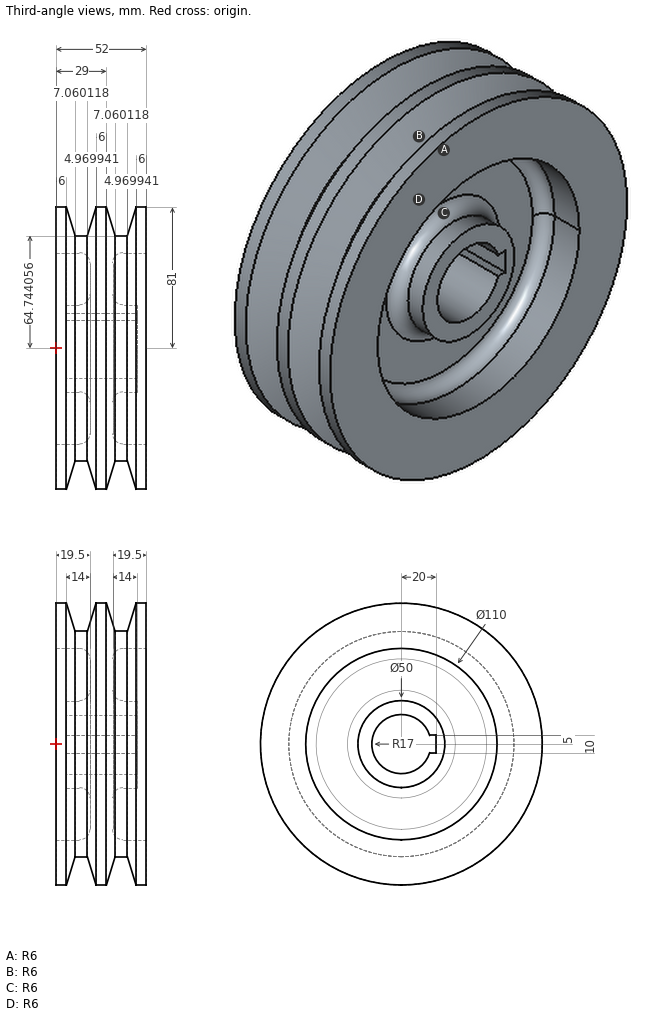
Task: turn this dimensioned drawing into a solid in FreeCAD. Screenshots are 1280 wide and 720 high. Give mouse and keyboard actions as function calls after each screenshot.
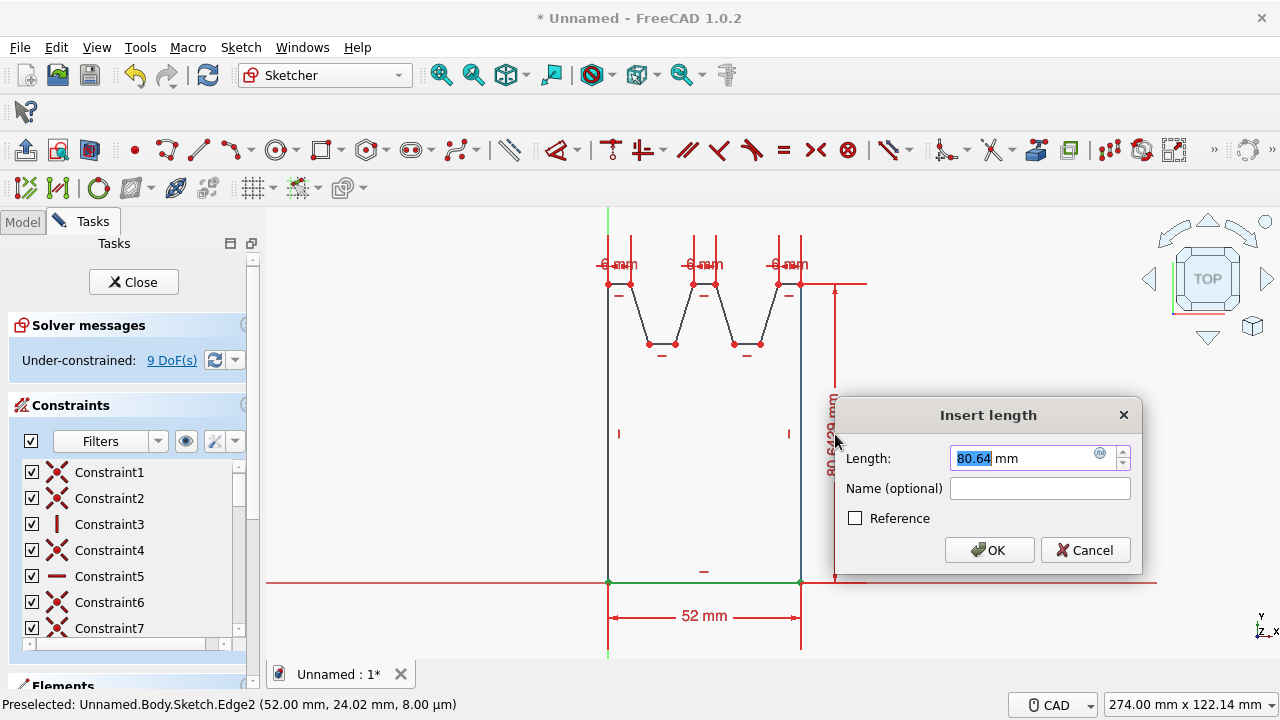
text(81)
key(Return)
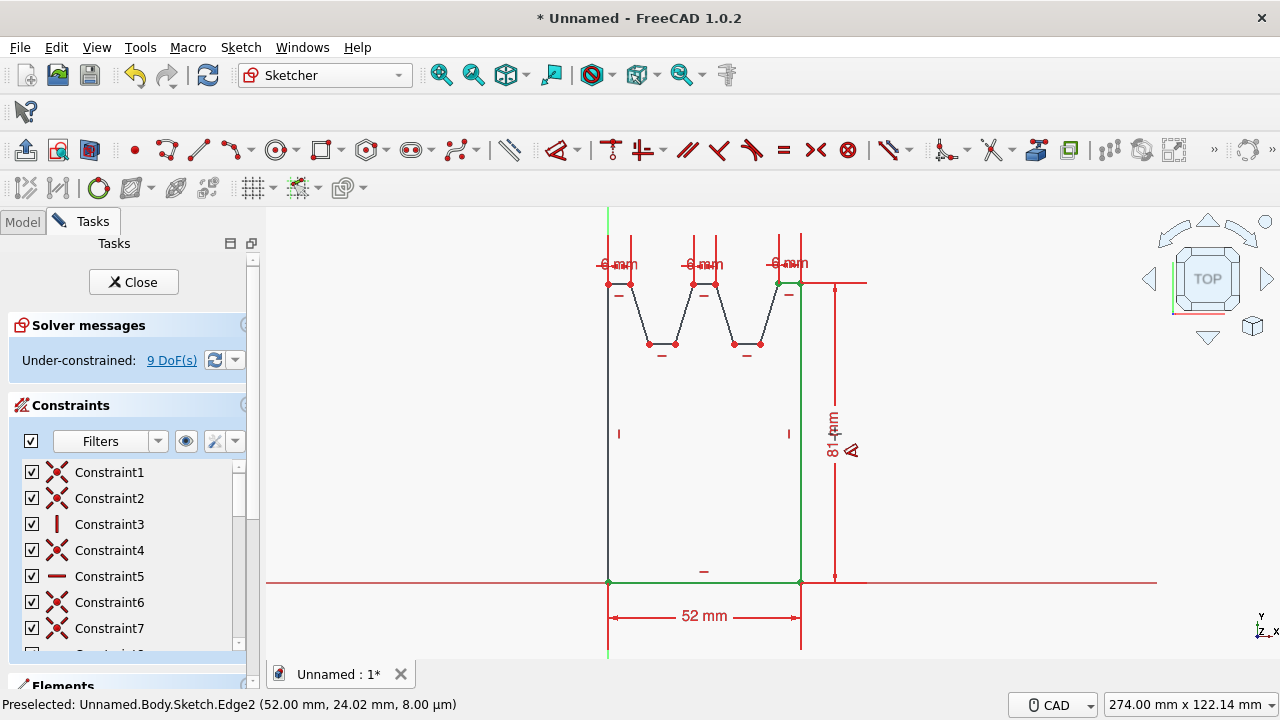
click(608, 374)
click(574, 434)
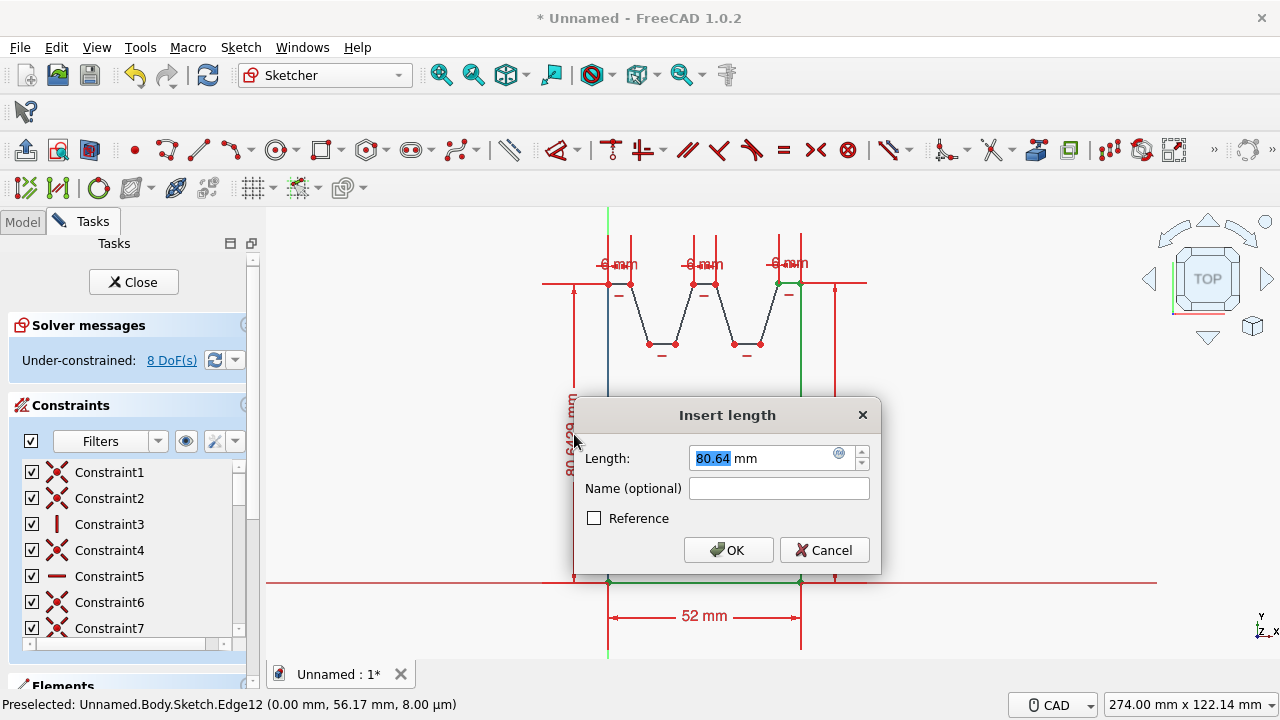
text(81)
key(Return)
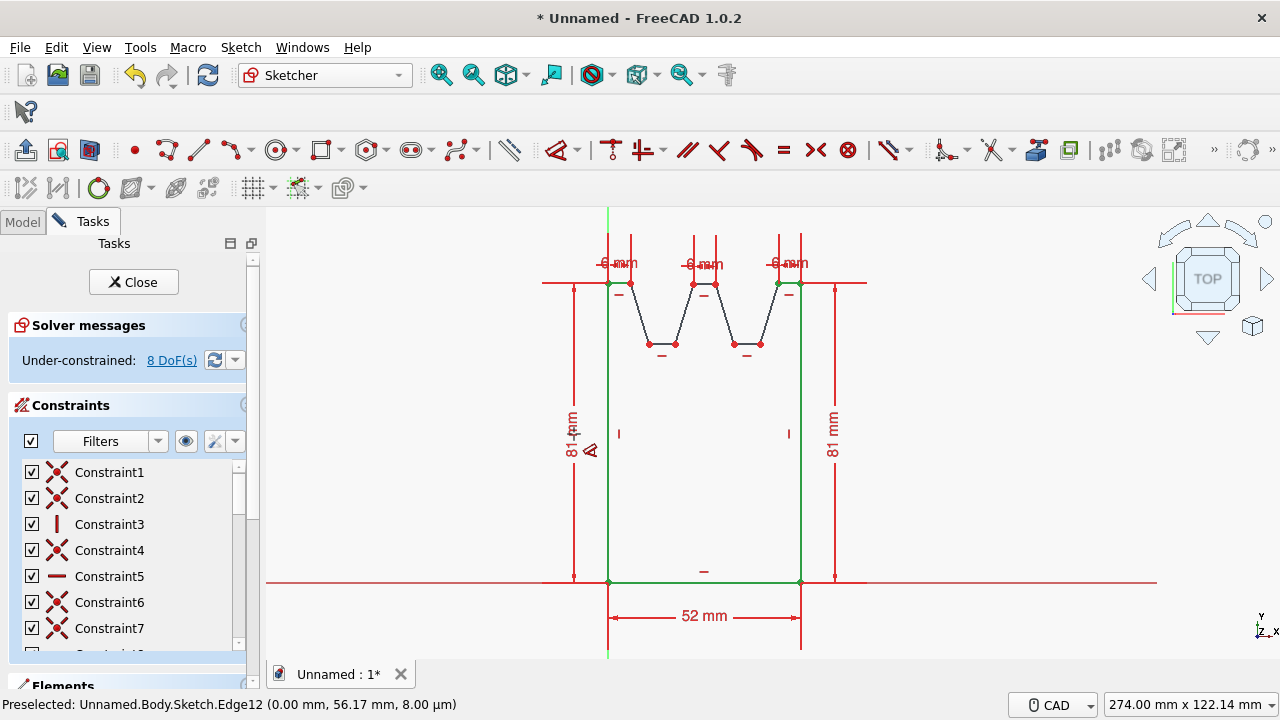
click(716, 284)
click(624, 617)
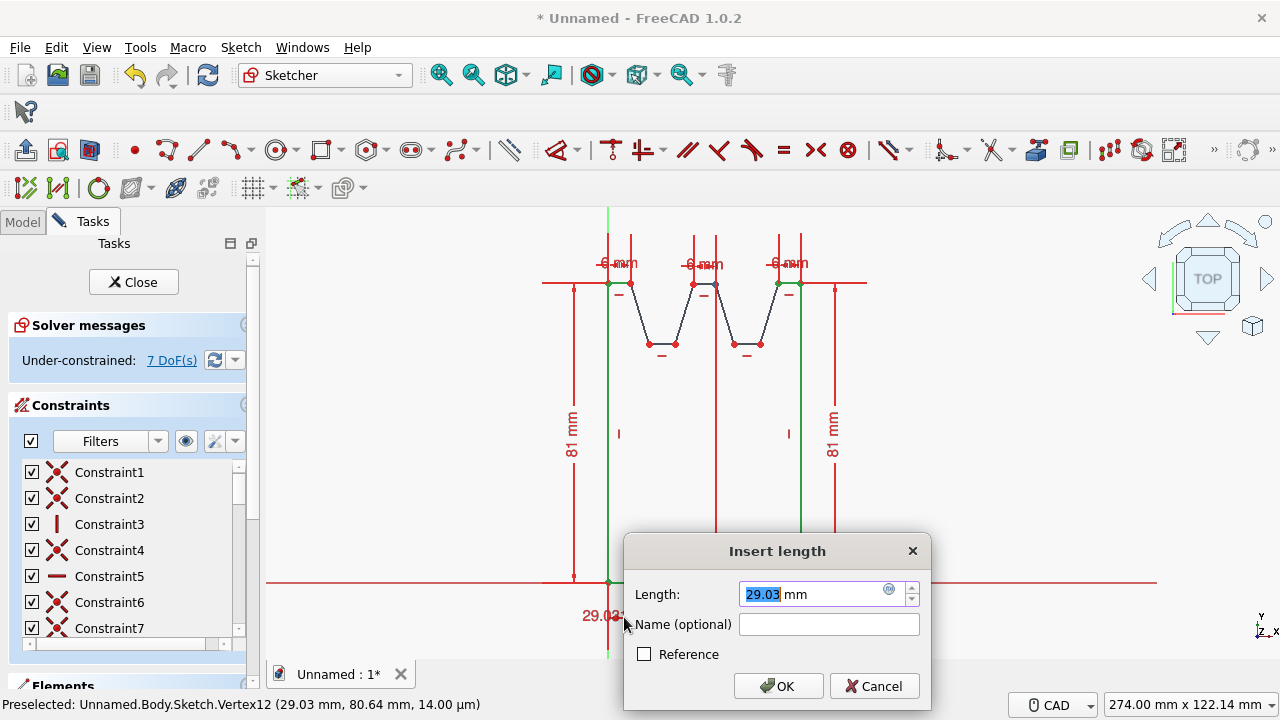
text(29)
key(Return)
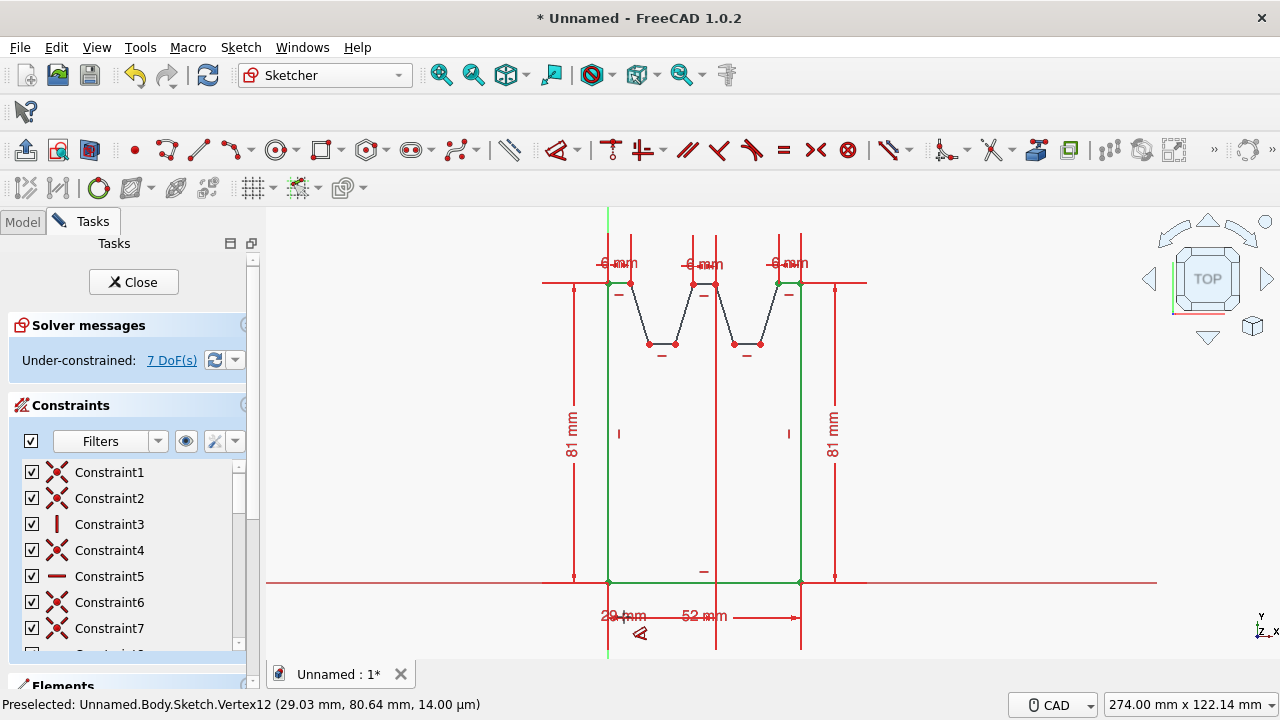
click(716, 284)
click(574, 365)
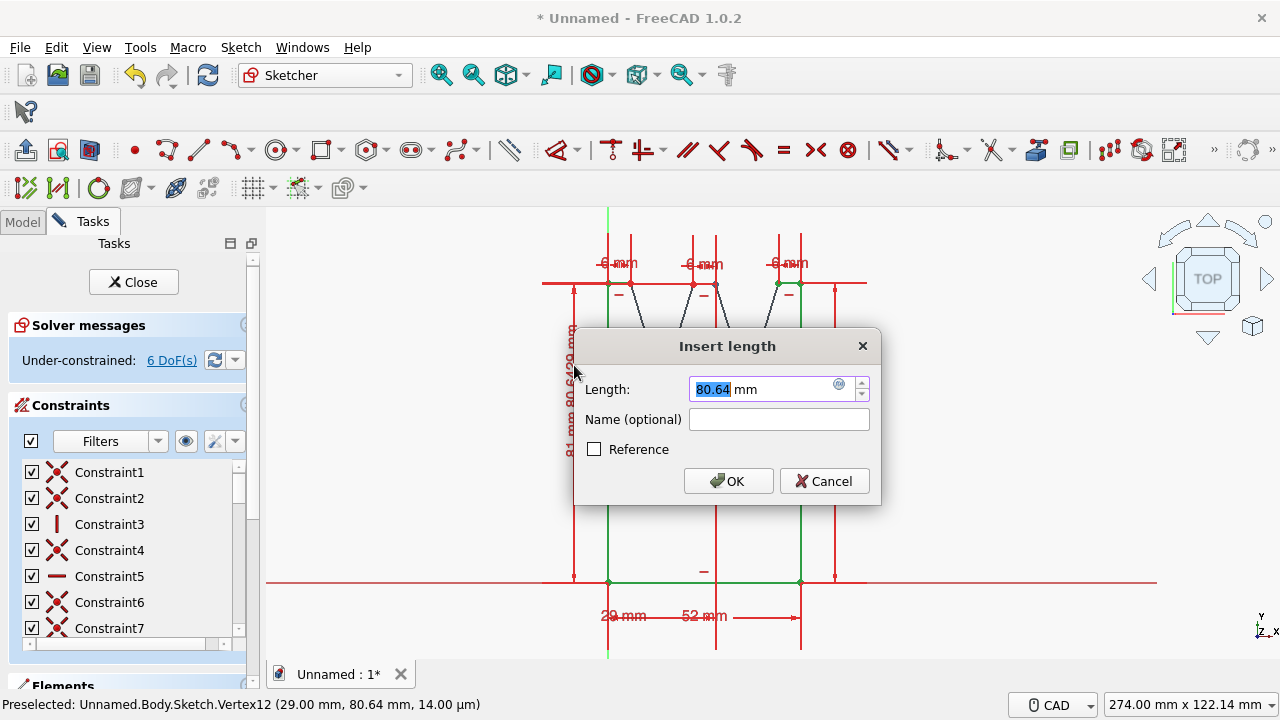
text(81)
key(Return)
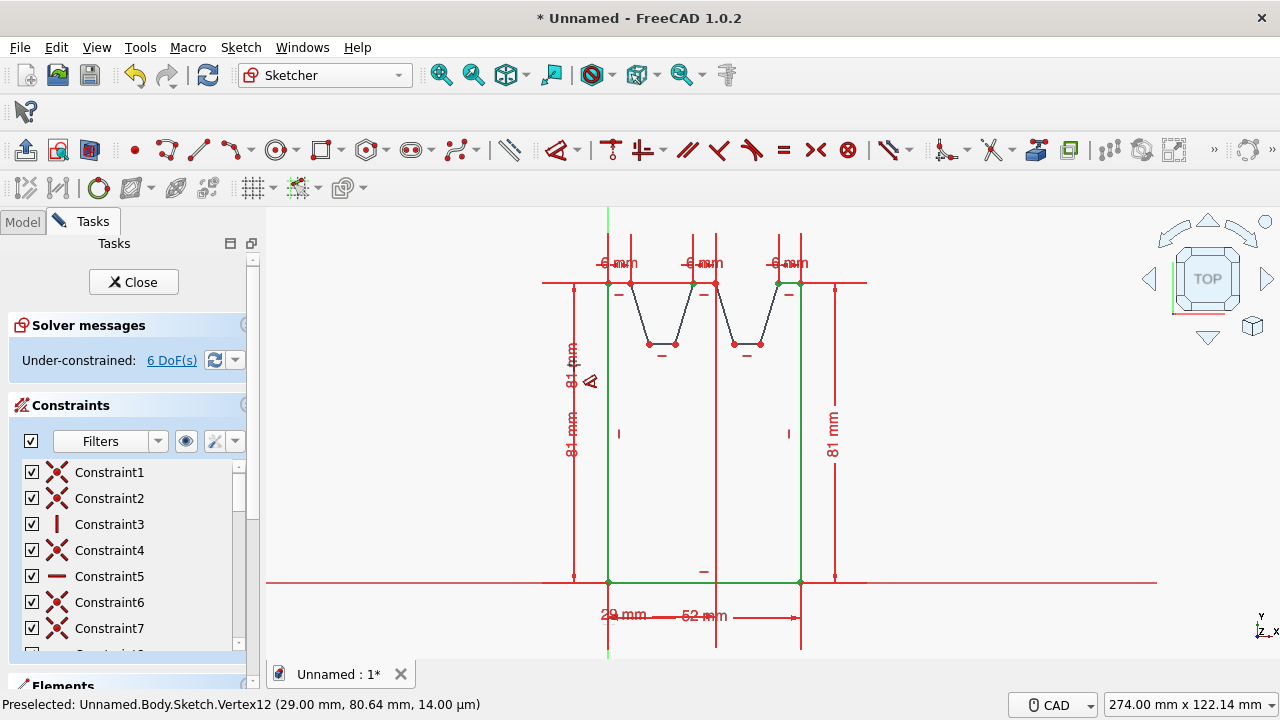
scroll(750, 344, up, 3)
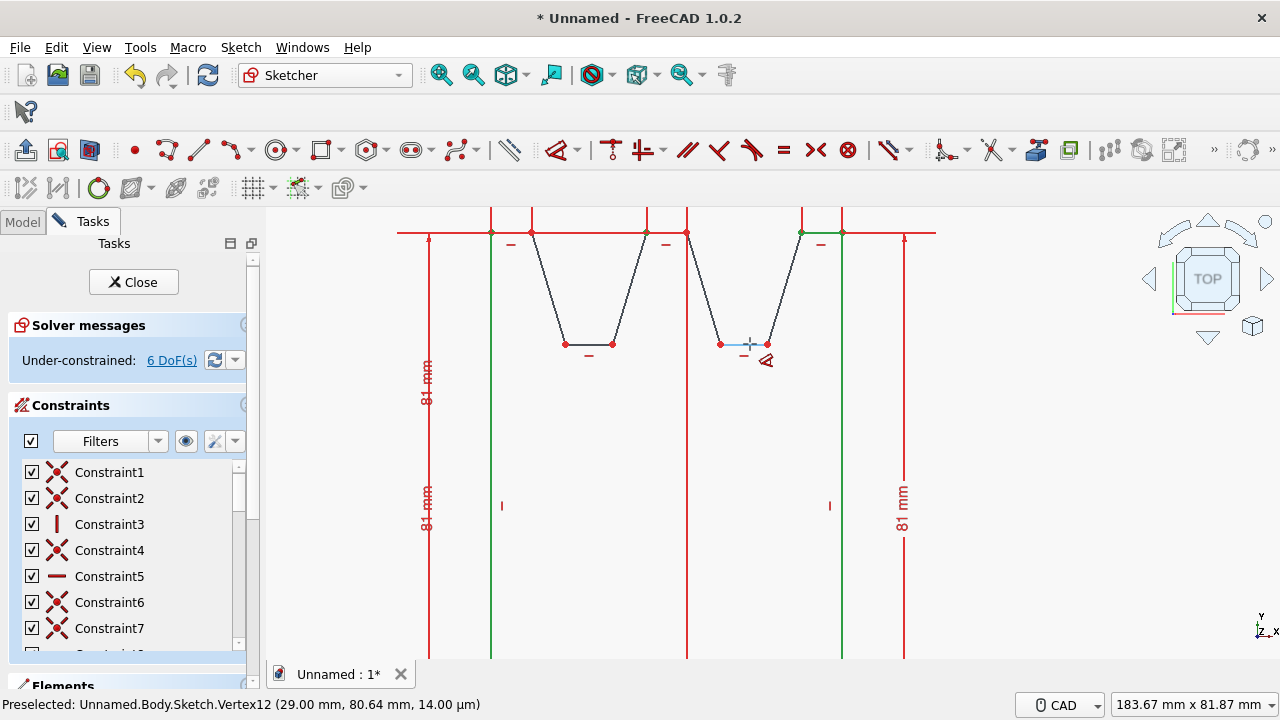
click(749, 345)
click(744, 311)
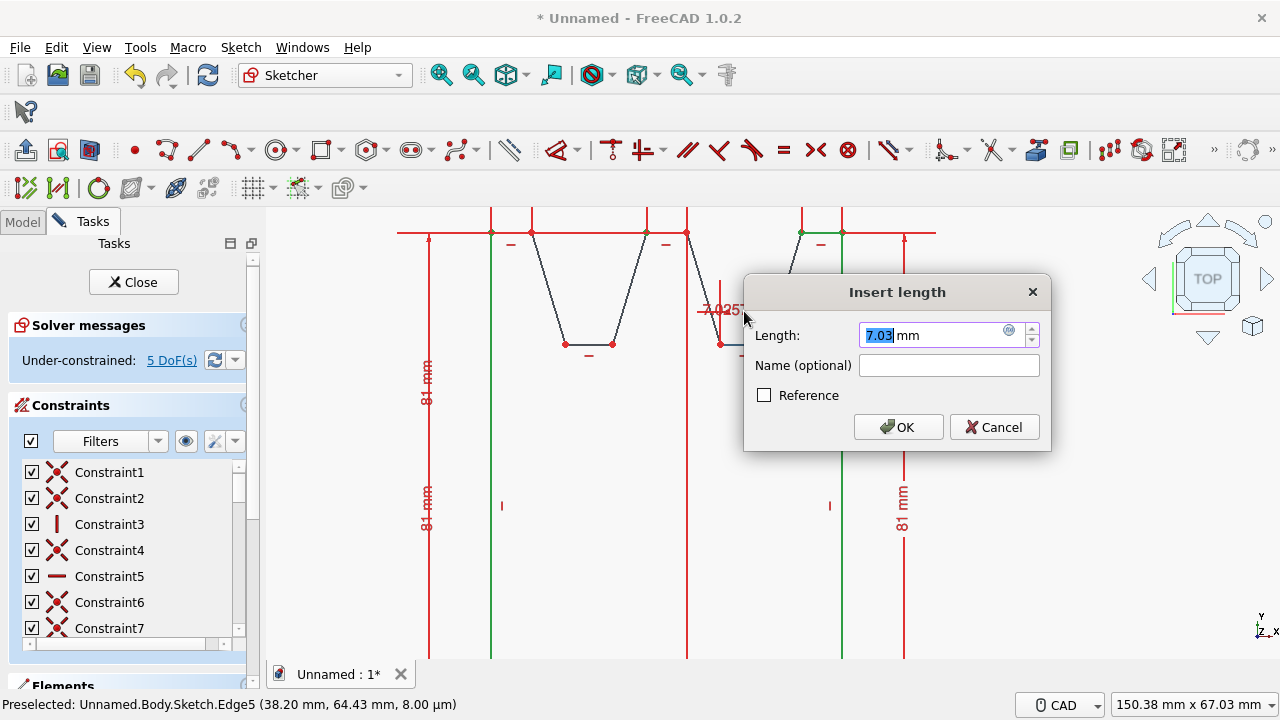
text(7.060118)
key(Return)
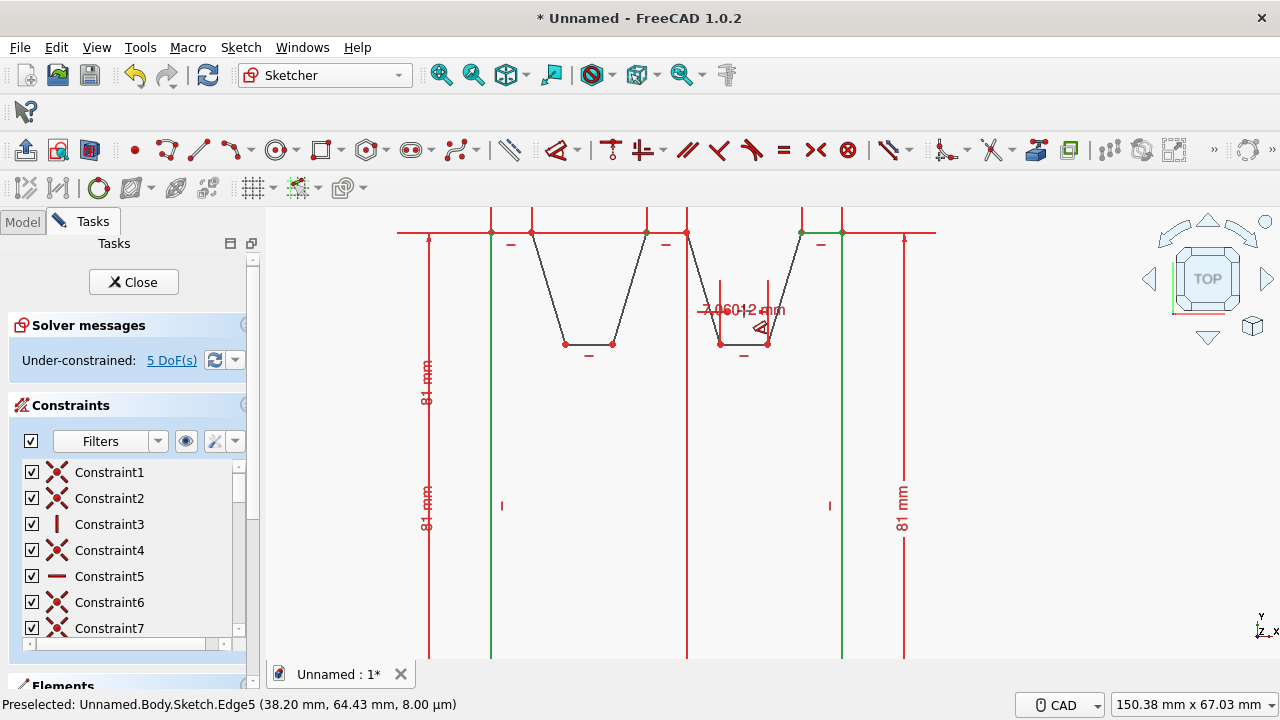
click(599, 345)
click(589, 311)